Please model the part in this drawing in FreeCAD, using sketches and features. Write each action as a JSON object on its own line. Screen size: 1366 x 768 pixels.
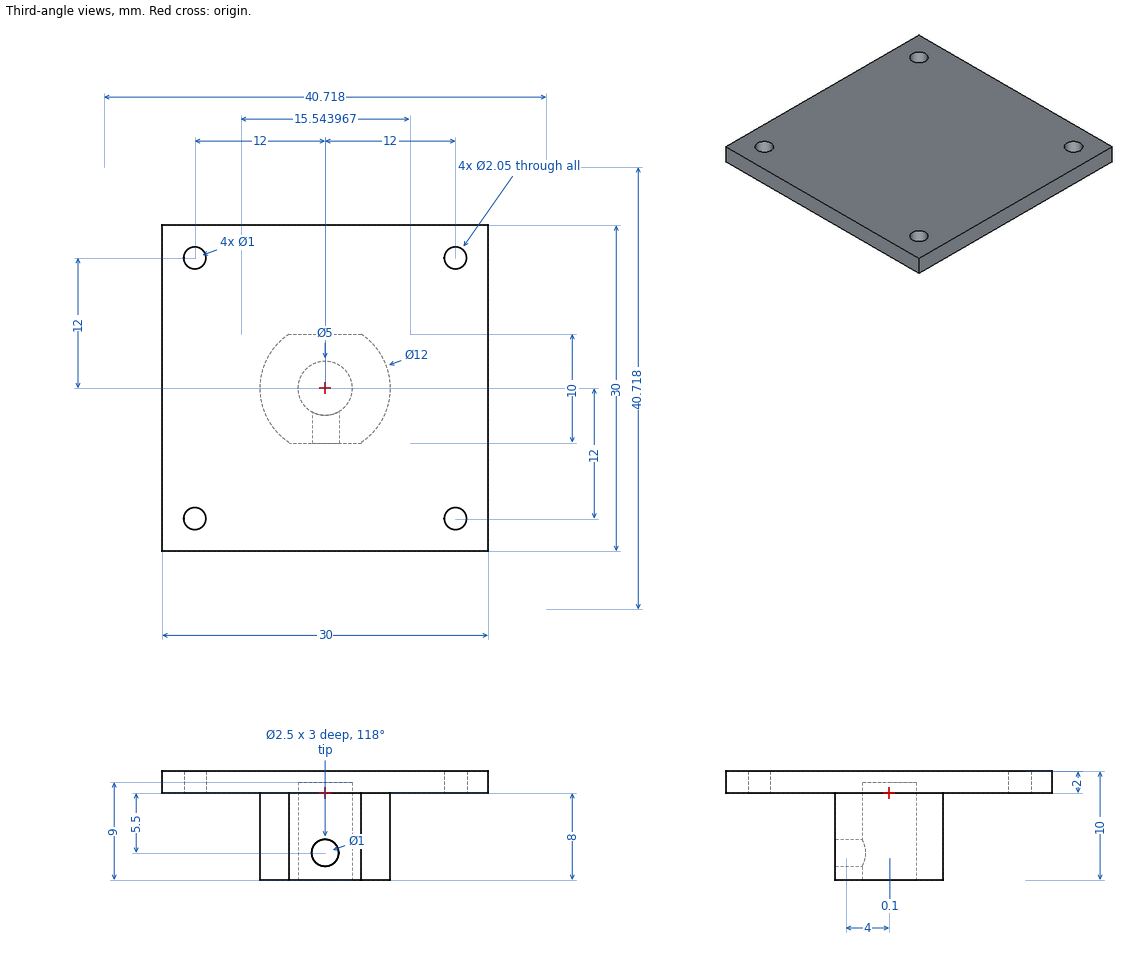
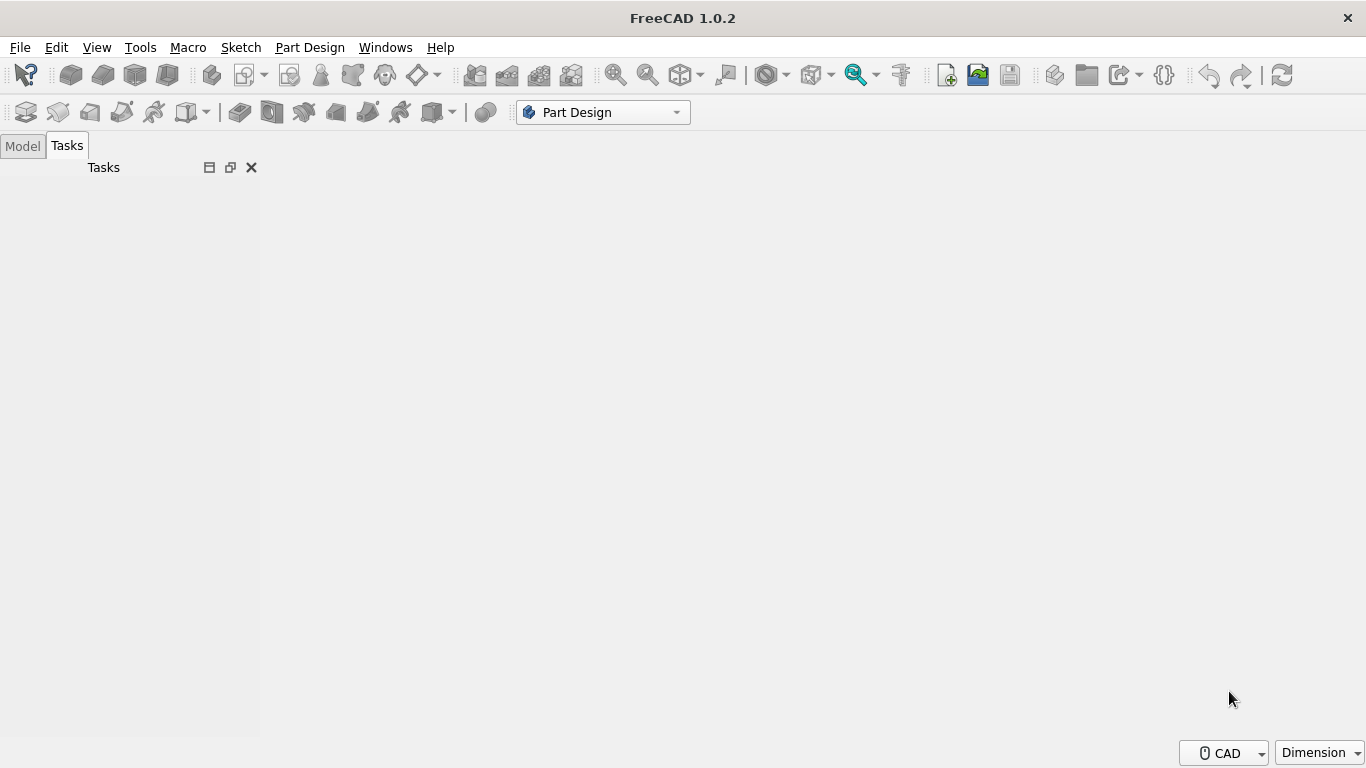
{"action": "key", "text": "ctrl+n"}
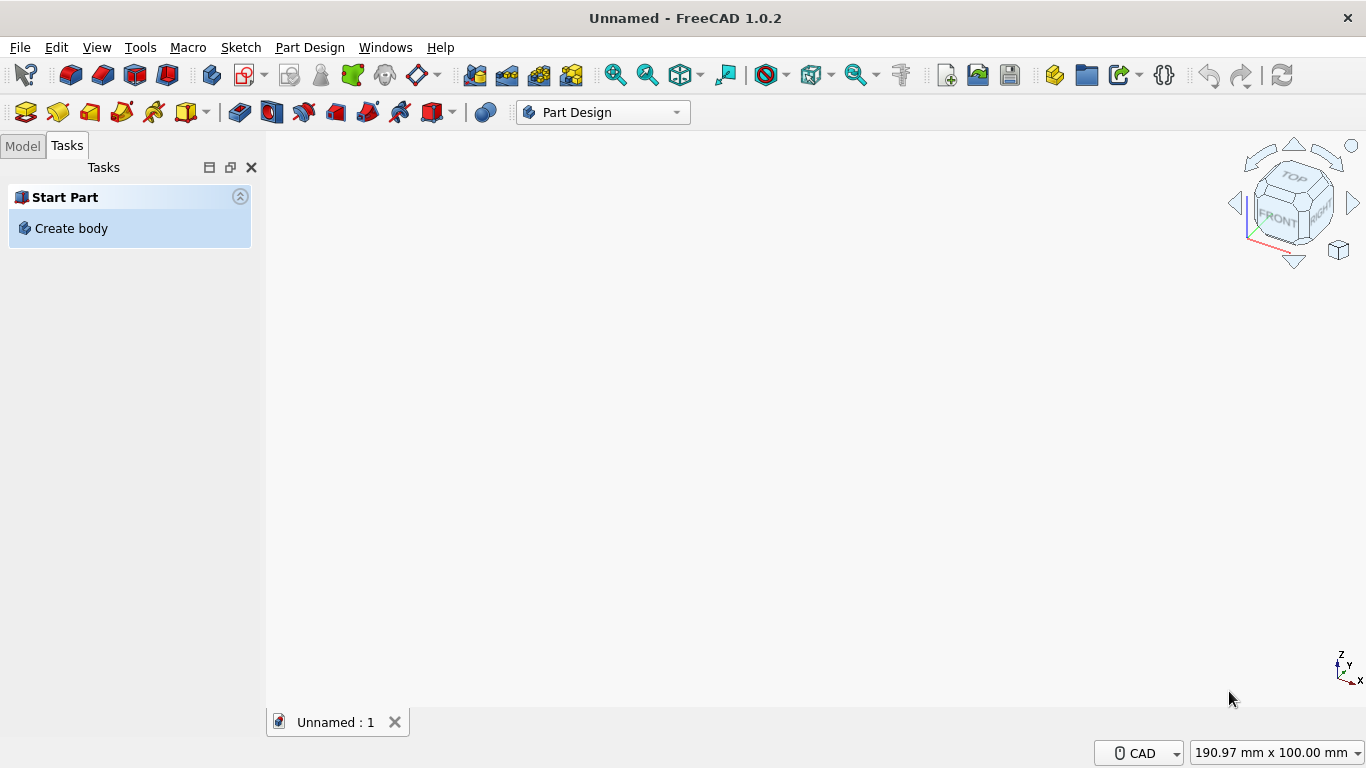
{"action": "left_click", "coordinate": [244, 76]}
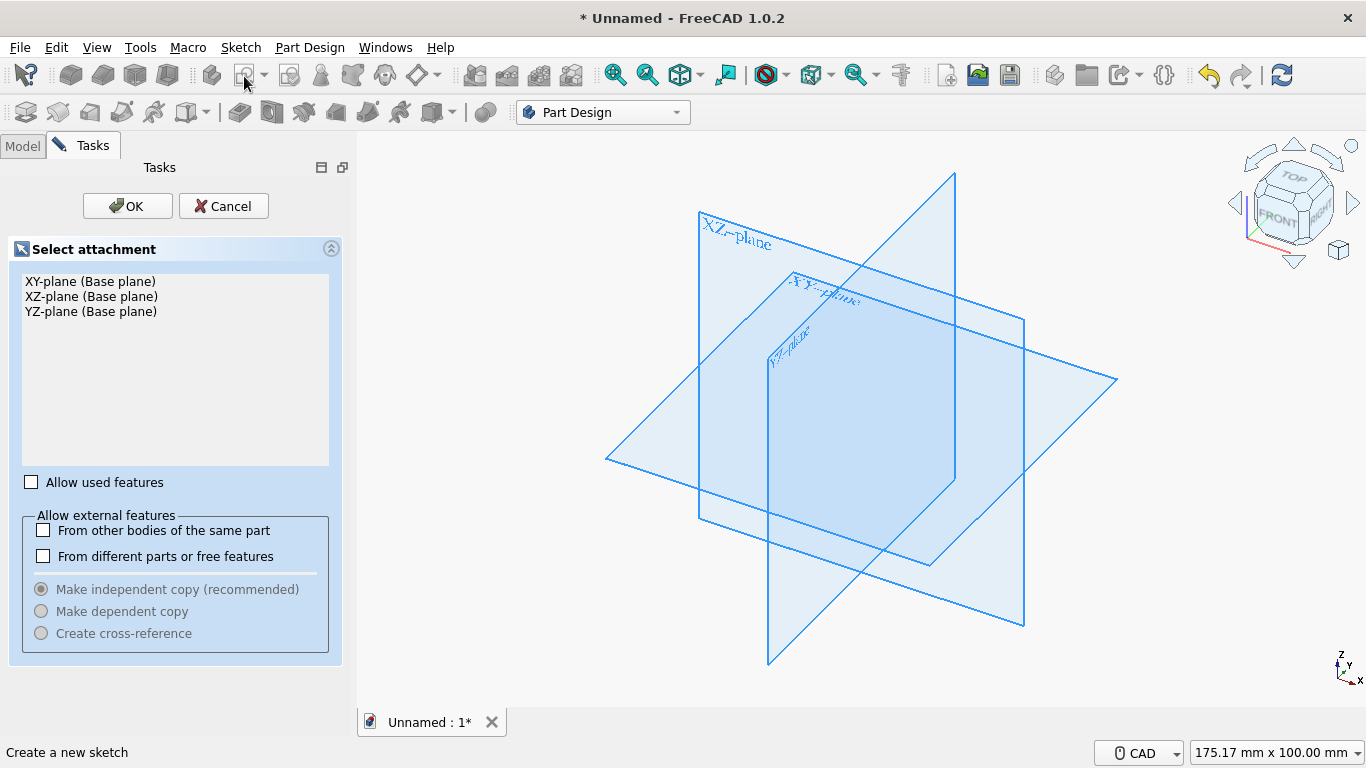
{"action": "left_click", "coordinate": [82, 282]}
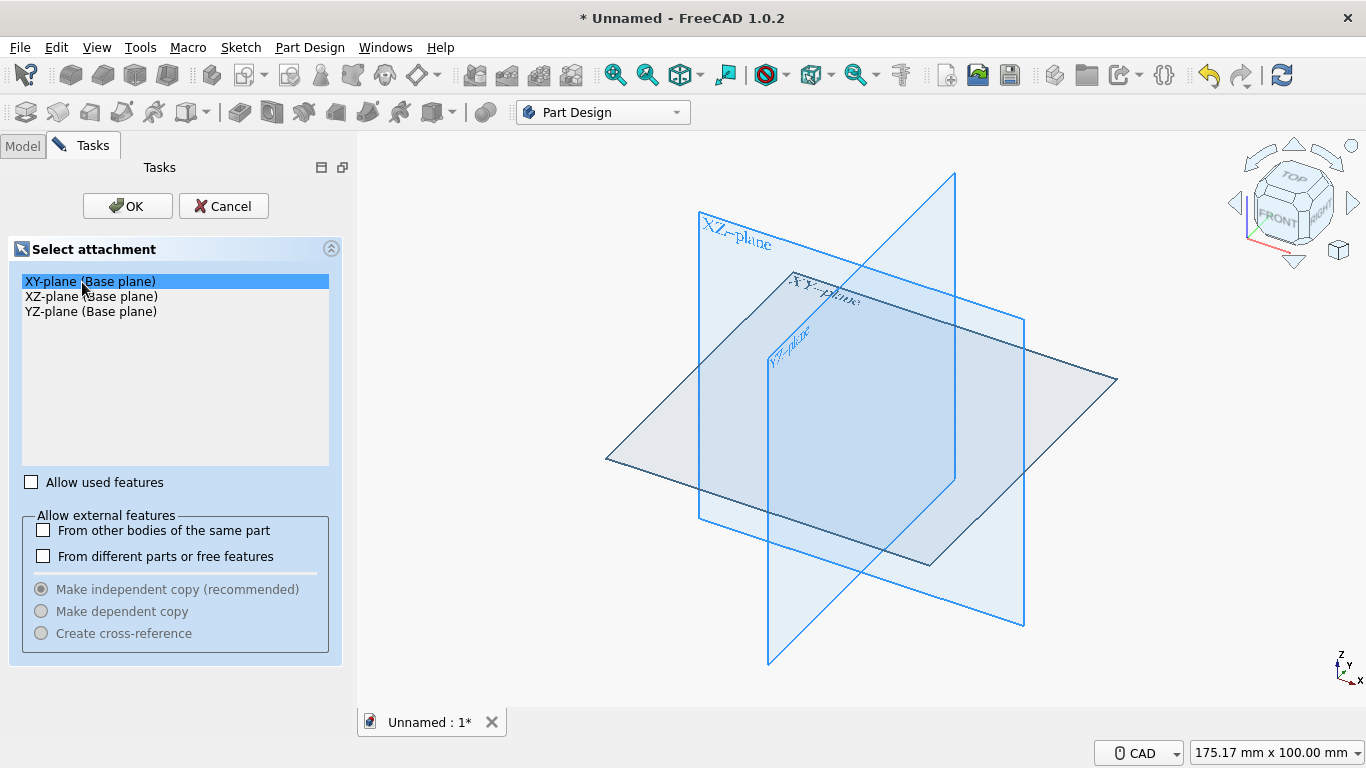
{"action": "left_click", "coordinate": [128, 206]}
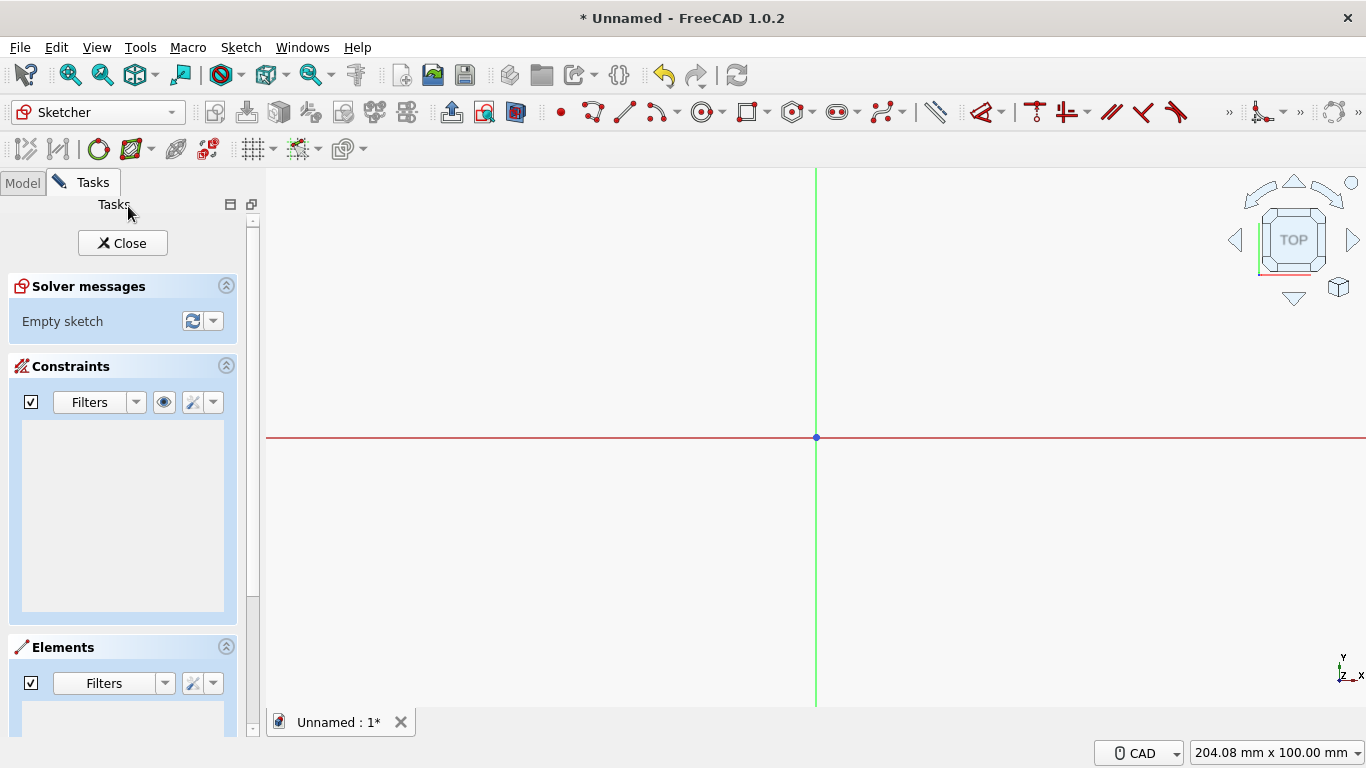
{"action": "scroll", "coordinate": [872, 438], "scroll_direction": "up", "scroll_amount": 4}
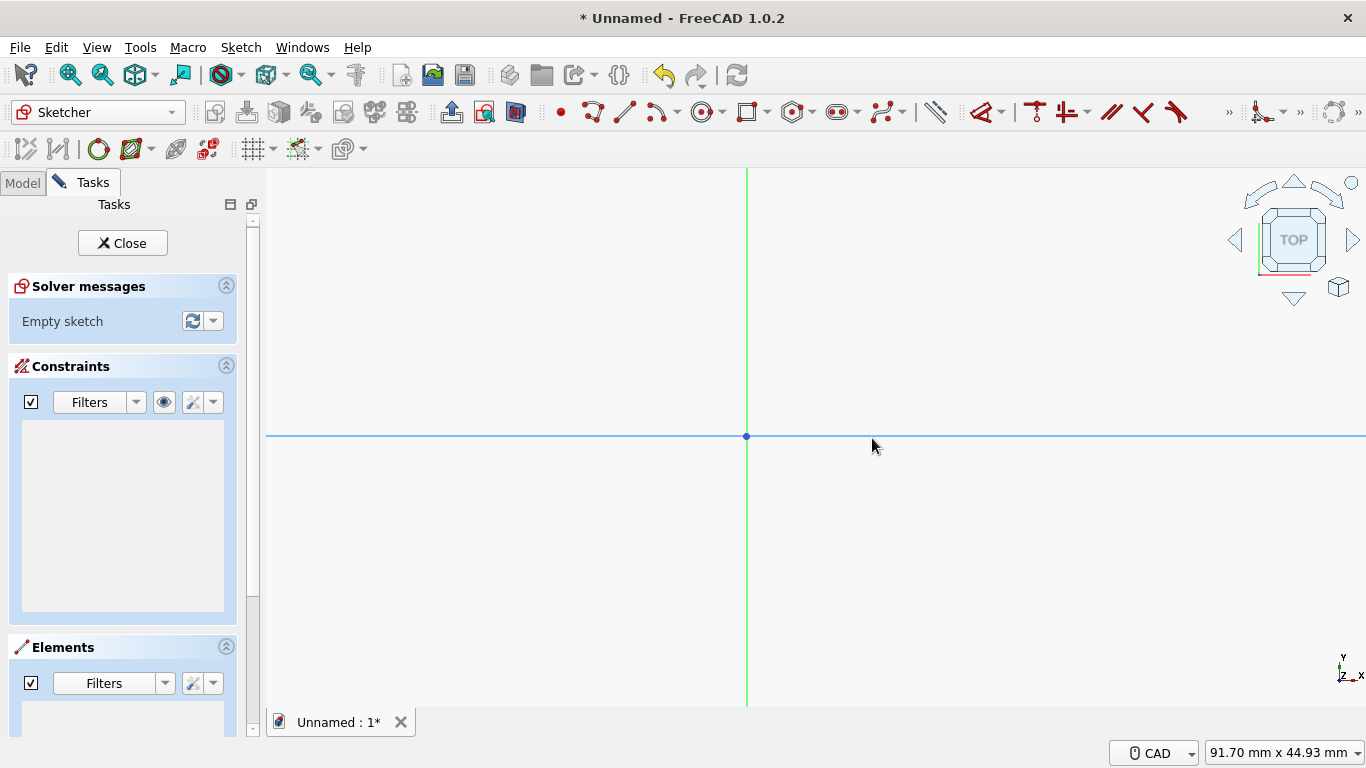
{"action": "left_click", "coordinate": [770, 112]}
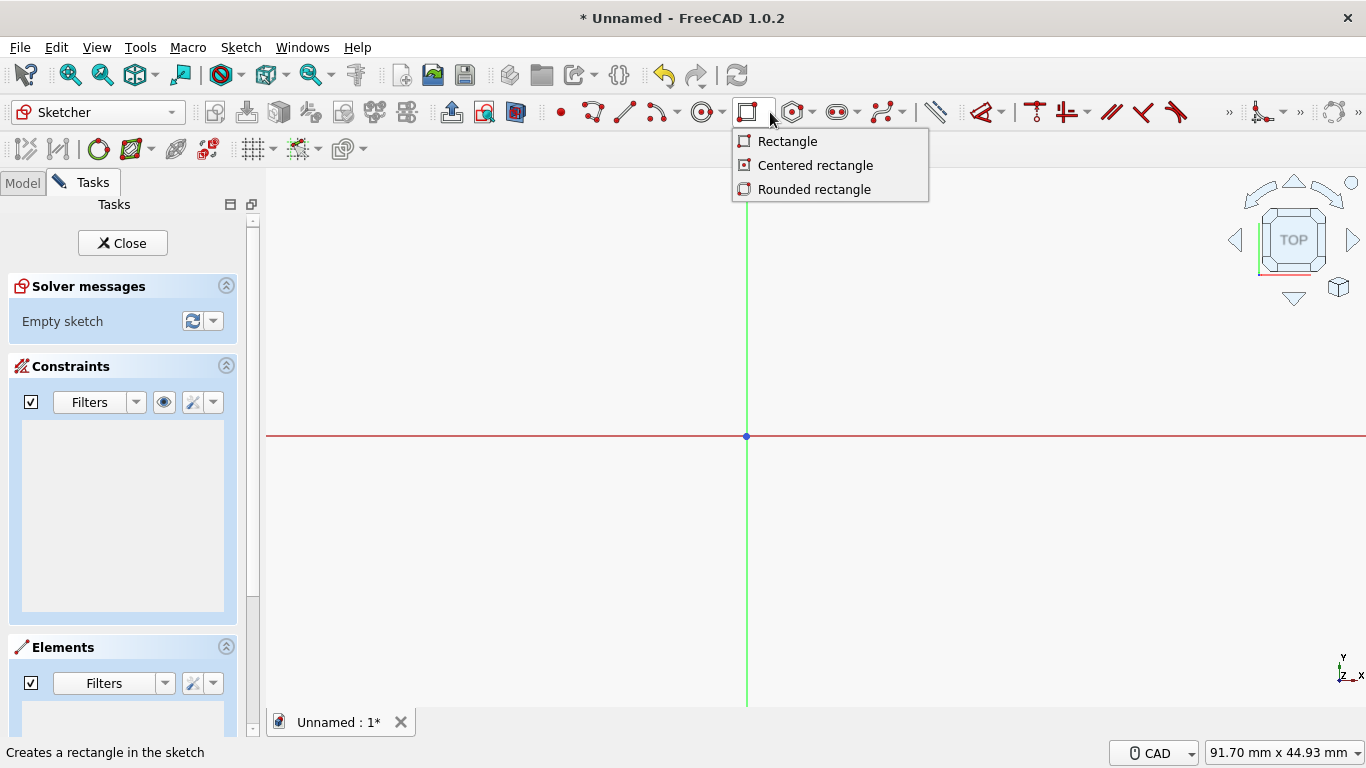
{"action": "left_click", "coordinate": [830, 165]}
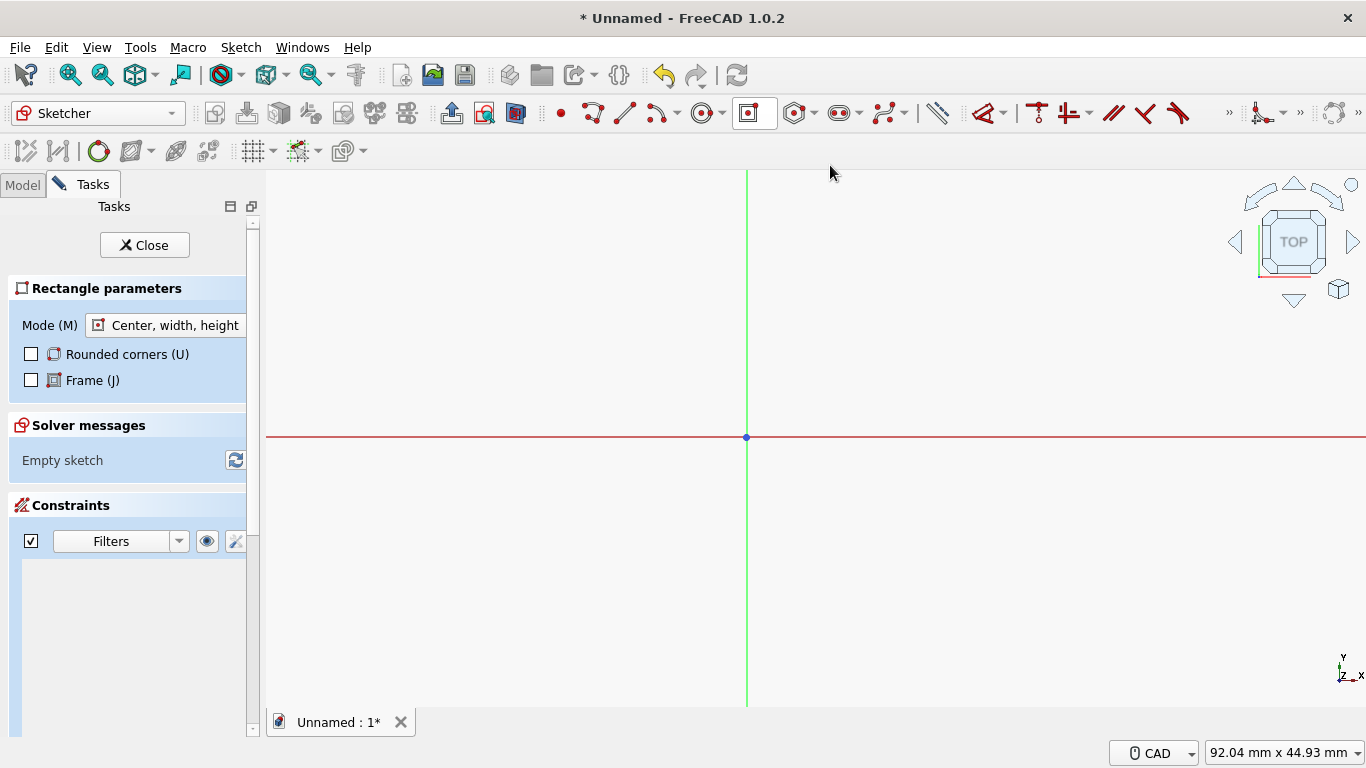
{"action": "left_click", "coordinate": [747, 437]}
{"action": "left_click", "coordinate": [926, 258]}
{"action": "key", "text": "Escape"}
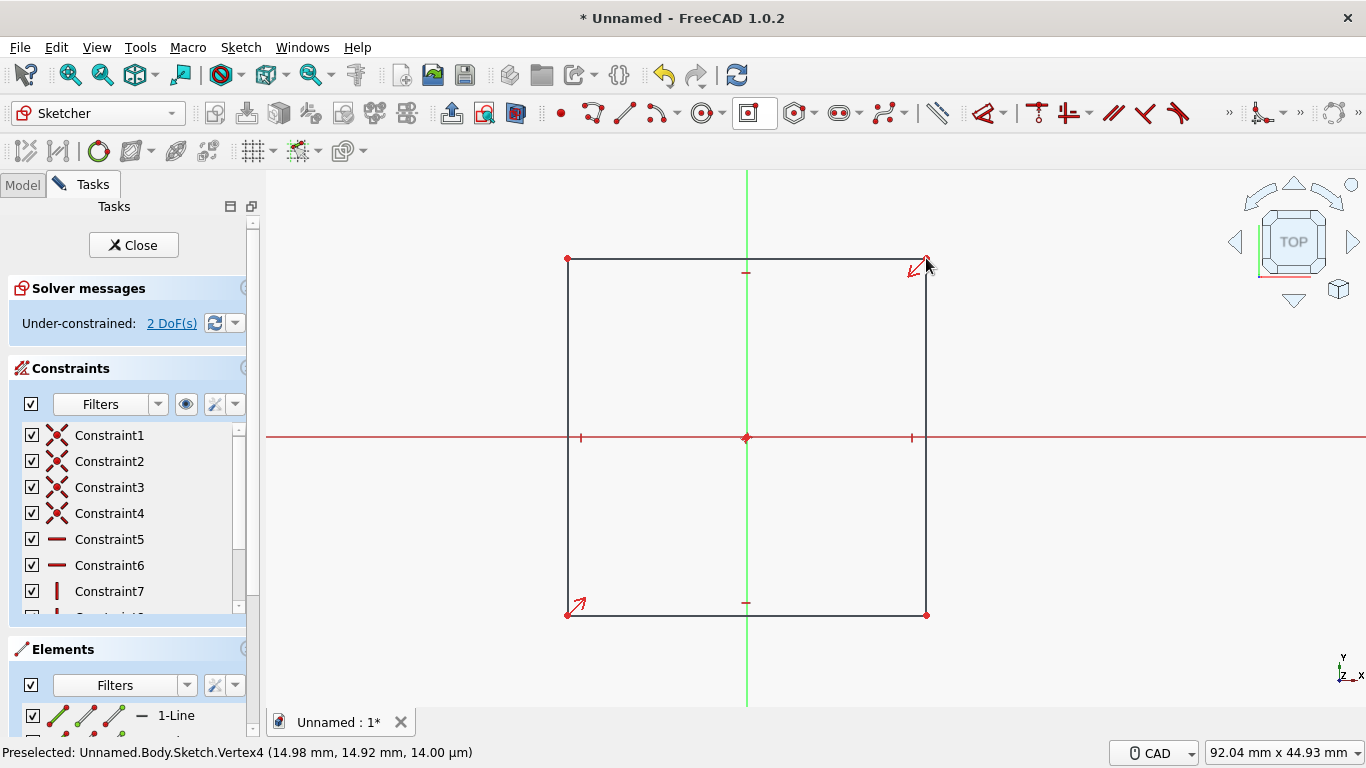
{"action": "key", "text": "d"}